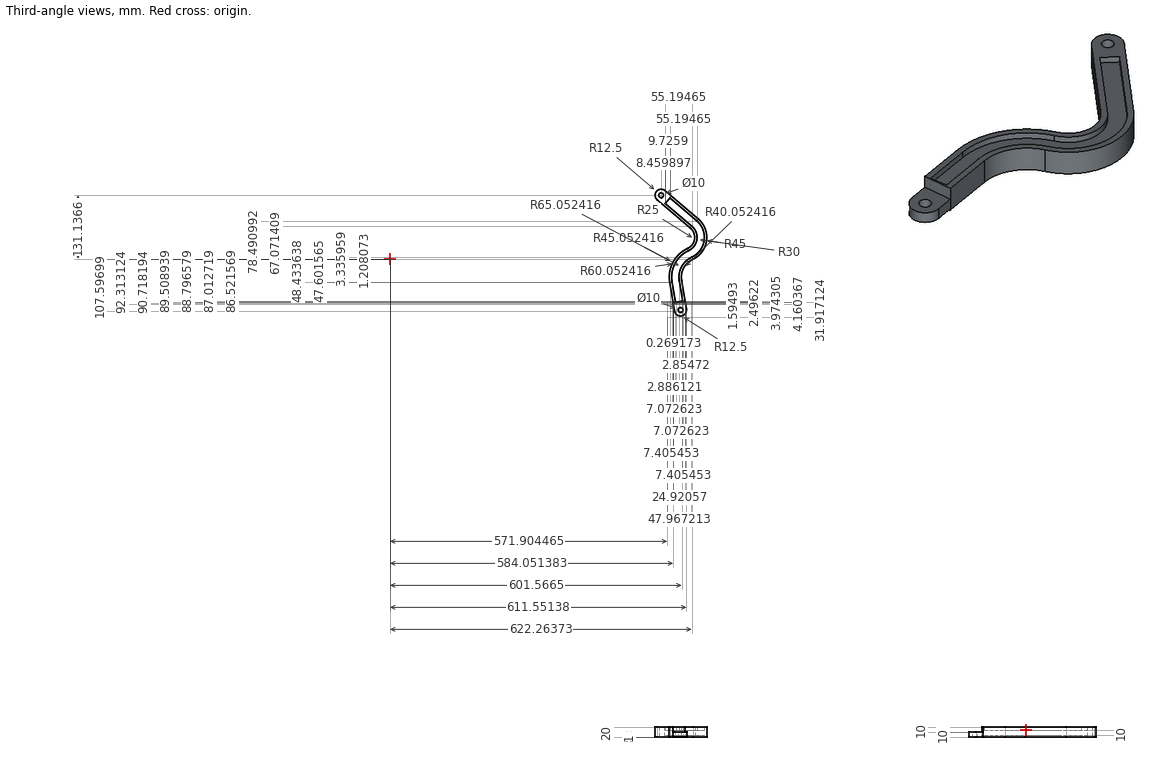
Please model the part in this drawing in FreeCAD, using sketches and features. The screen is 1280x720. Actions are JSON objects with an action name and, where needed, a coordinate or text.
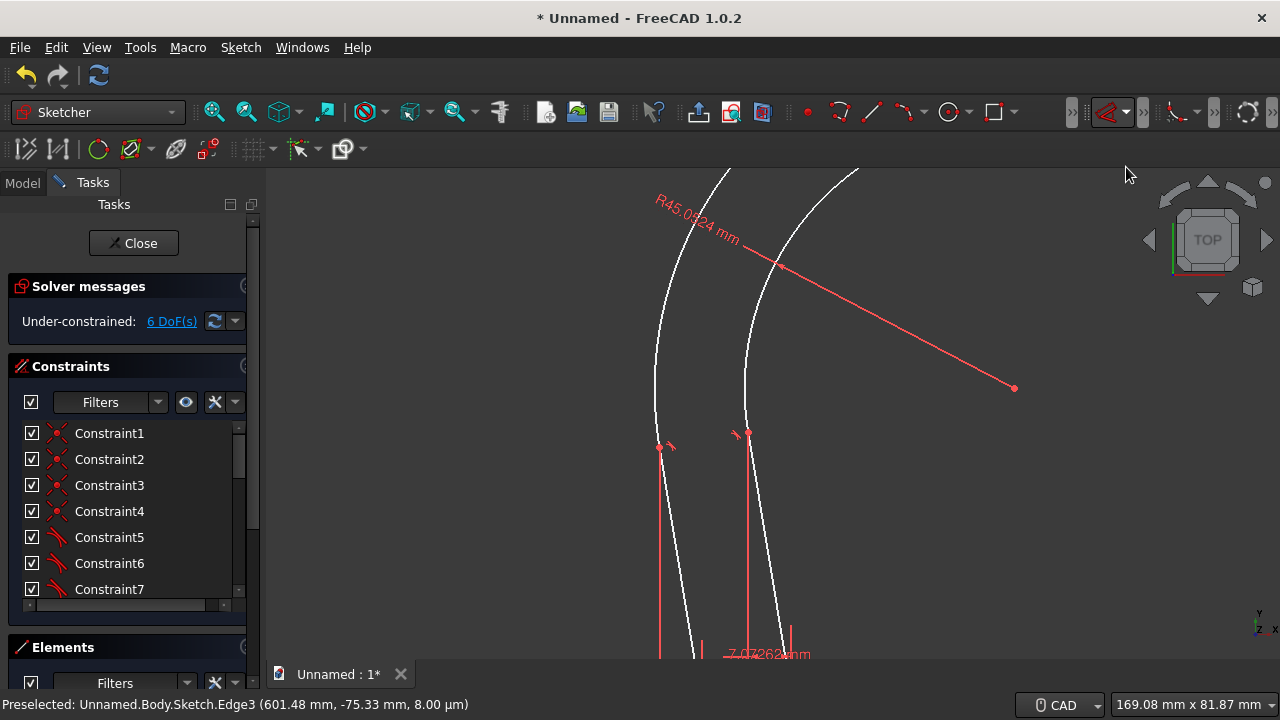
{"action": "scroll", "coordinate": [668, 530], "scroll_direction": "down", "scroll_amount": 7}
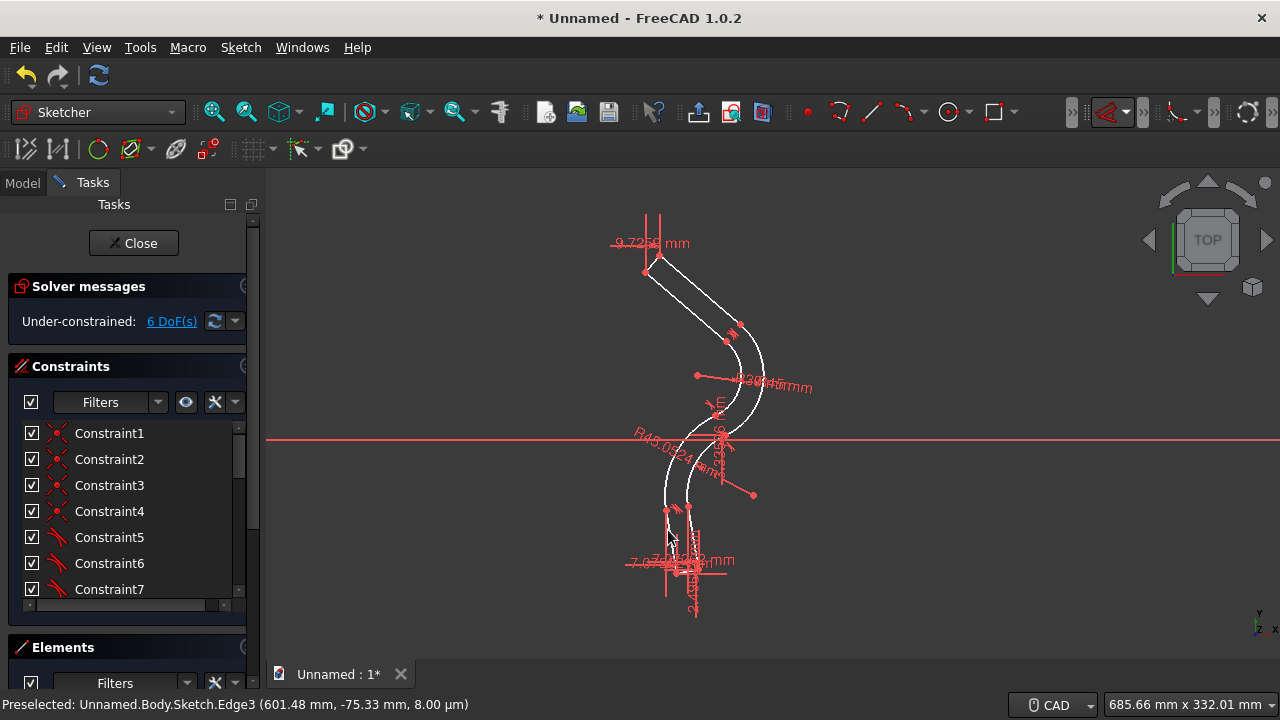
{"action": "left_click", "coordinate": [716, 304]}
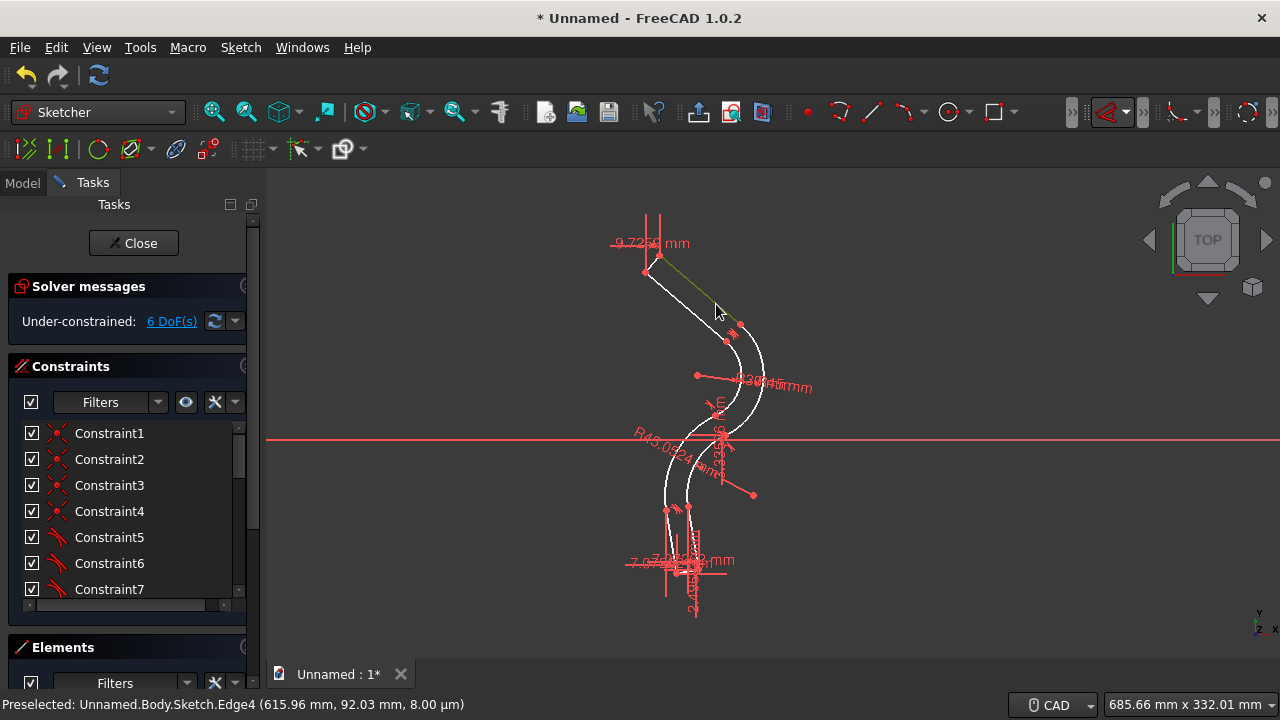
{"action": "key", "text": "l"}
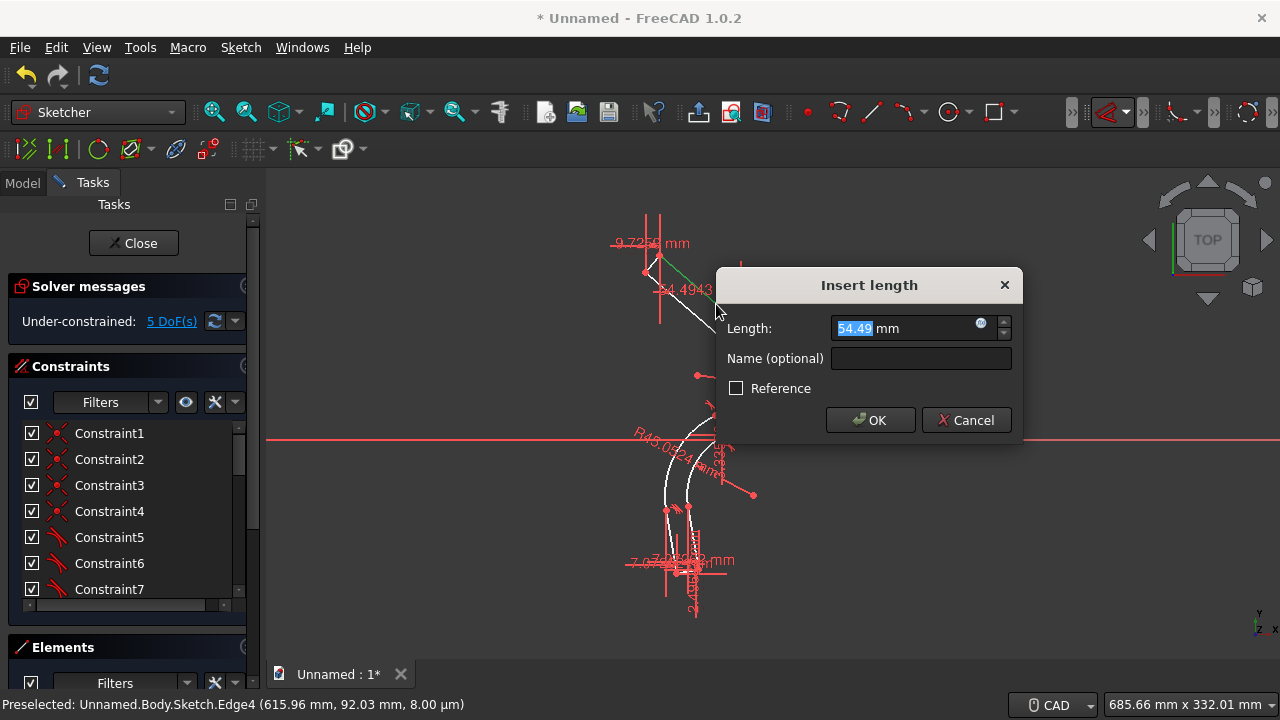
{"action": "type", "text": "55.19465"}
{"action": "key", "text": "Return"}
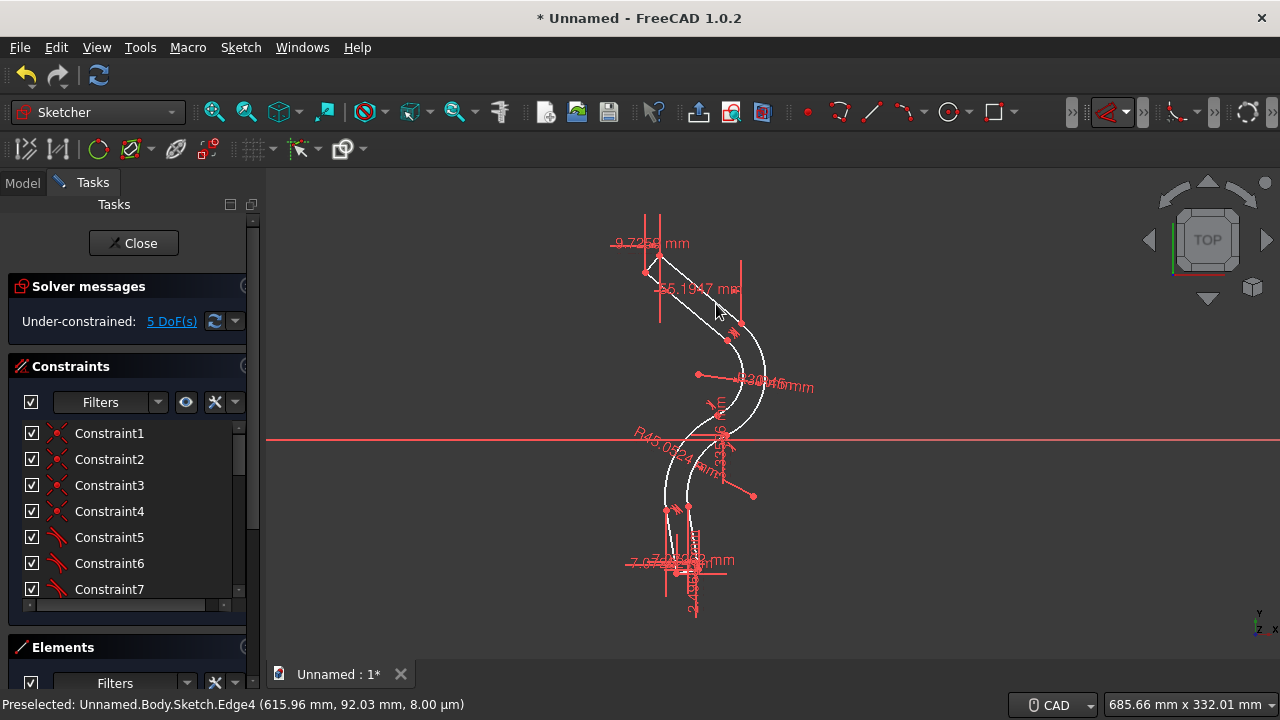
{"action": "left_click", "coordinate": [703, 320]}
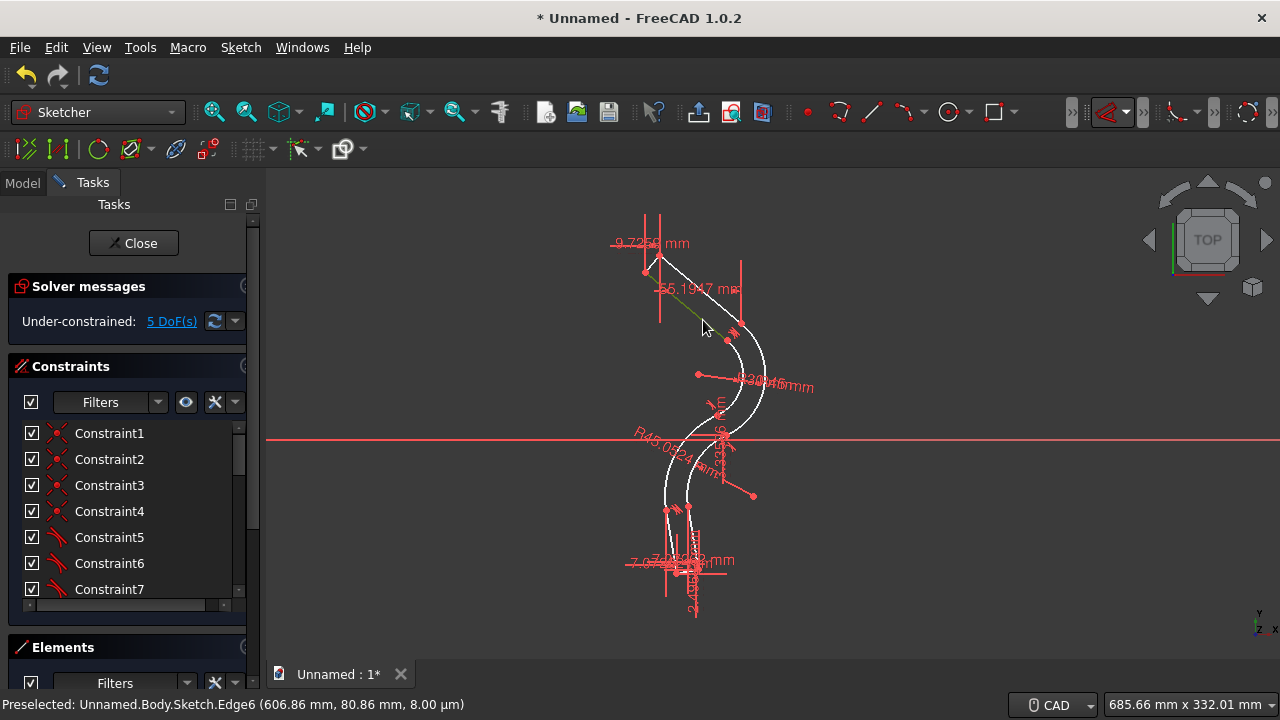
{"action": "left_click", "coordinate": [1128, 112]}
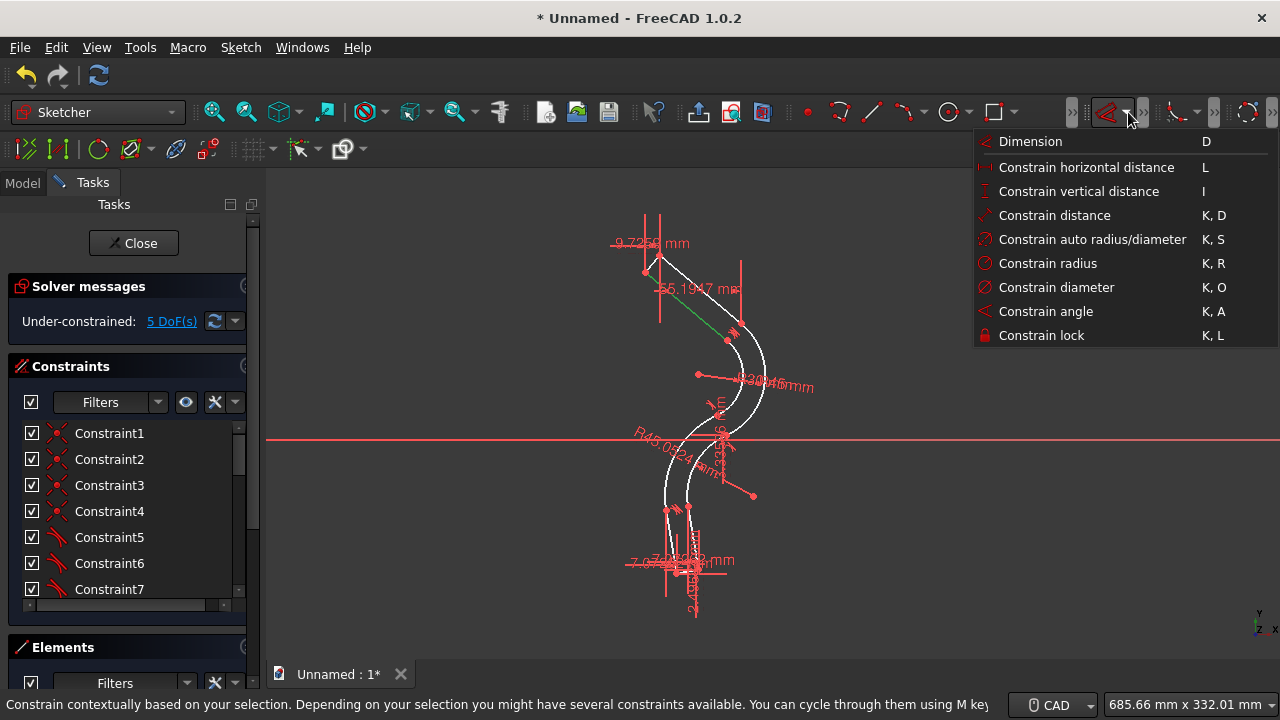
{"action": "left_click", "coordinate": [1126, 167]}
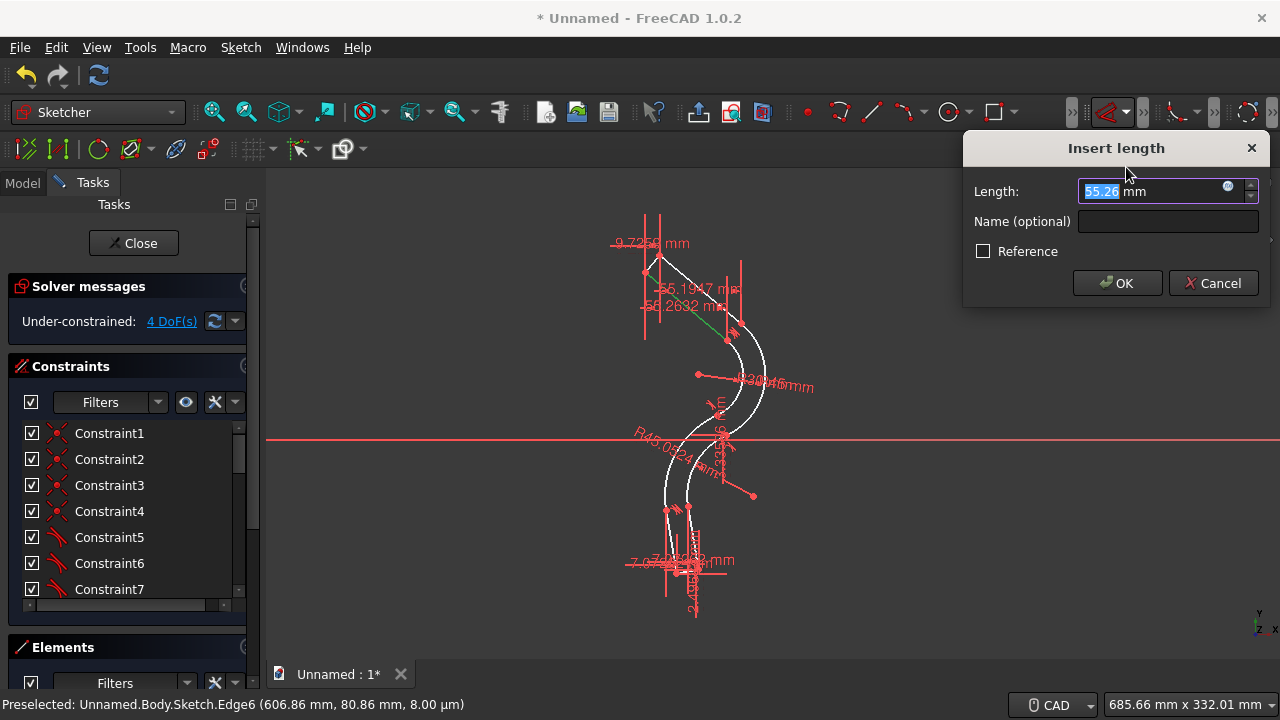
{"action": "type", "text": "55.19465"}
{"action": "key", "text": "Return"}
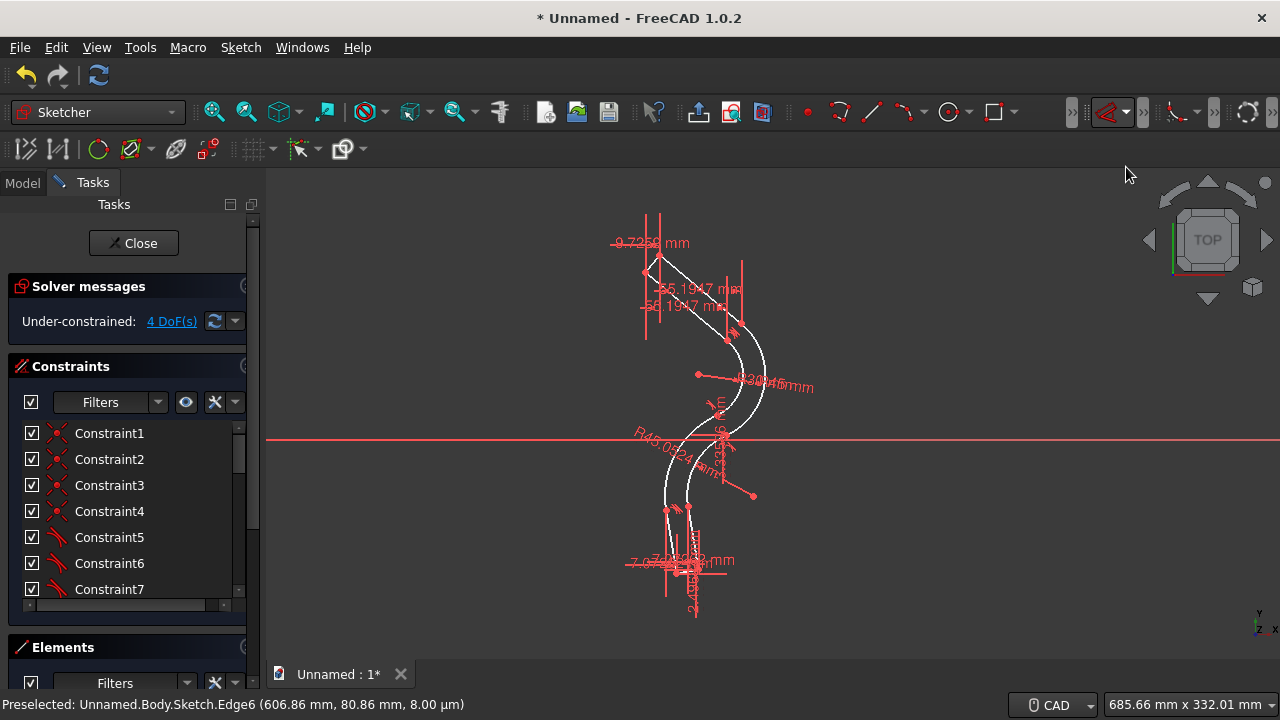
{"action": "left_click", "coordinate": [666, 511]}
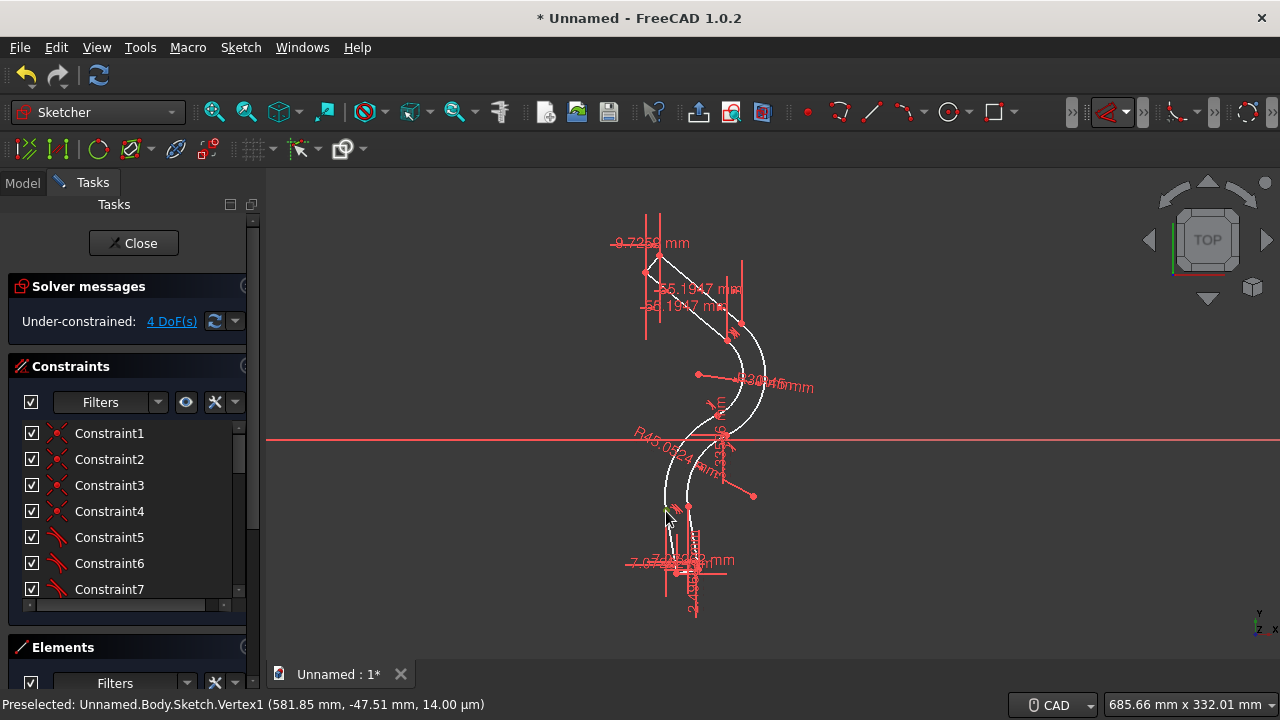
{"action": "key", "text": "i"}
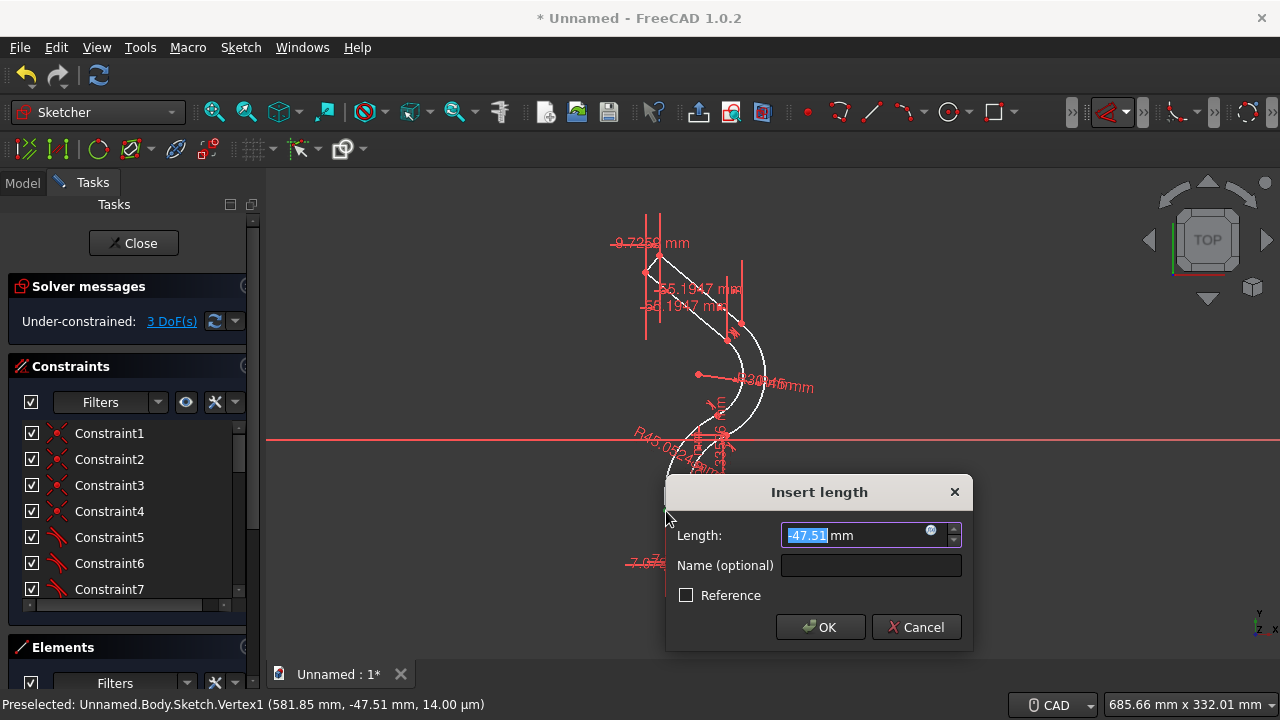
{"action": "type", "text": "-47.601565"}
{"action": "key", "text": "Return"}